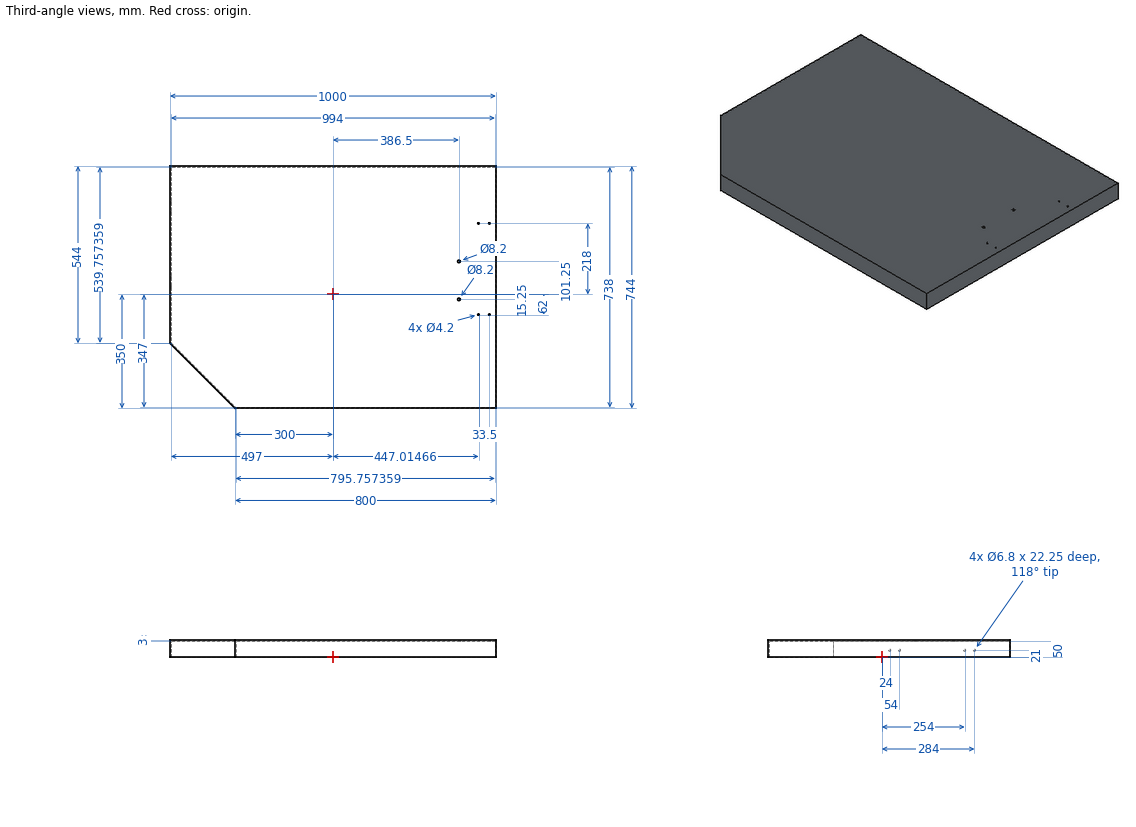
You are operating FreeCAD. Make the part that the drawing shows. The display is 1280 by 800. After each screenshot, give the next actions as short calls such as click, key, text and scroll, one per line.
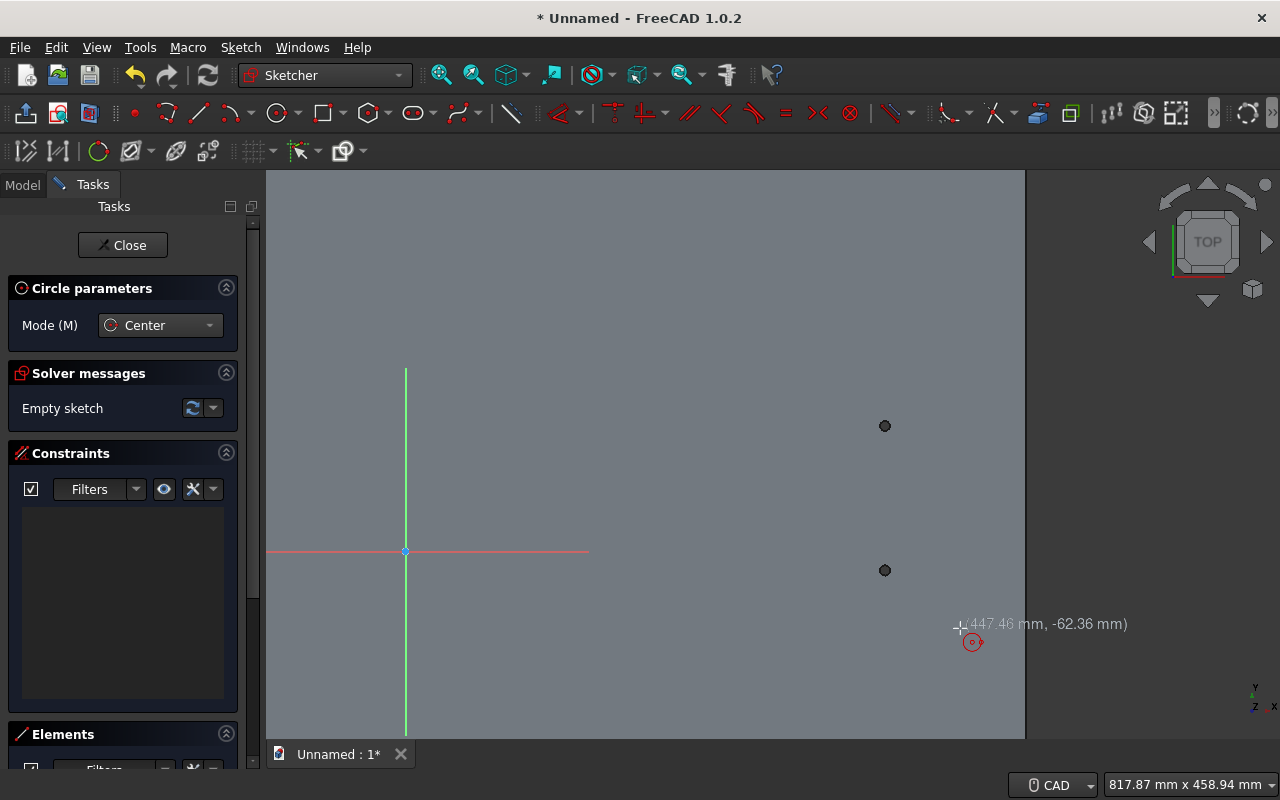
click(960, 628)
move(962, 627)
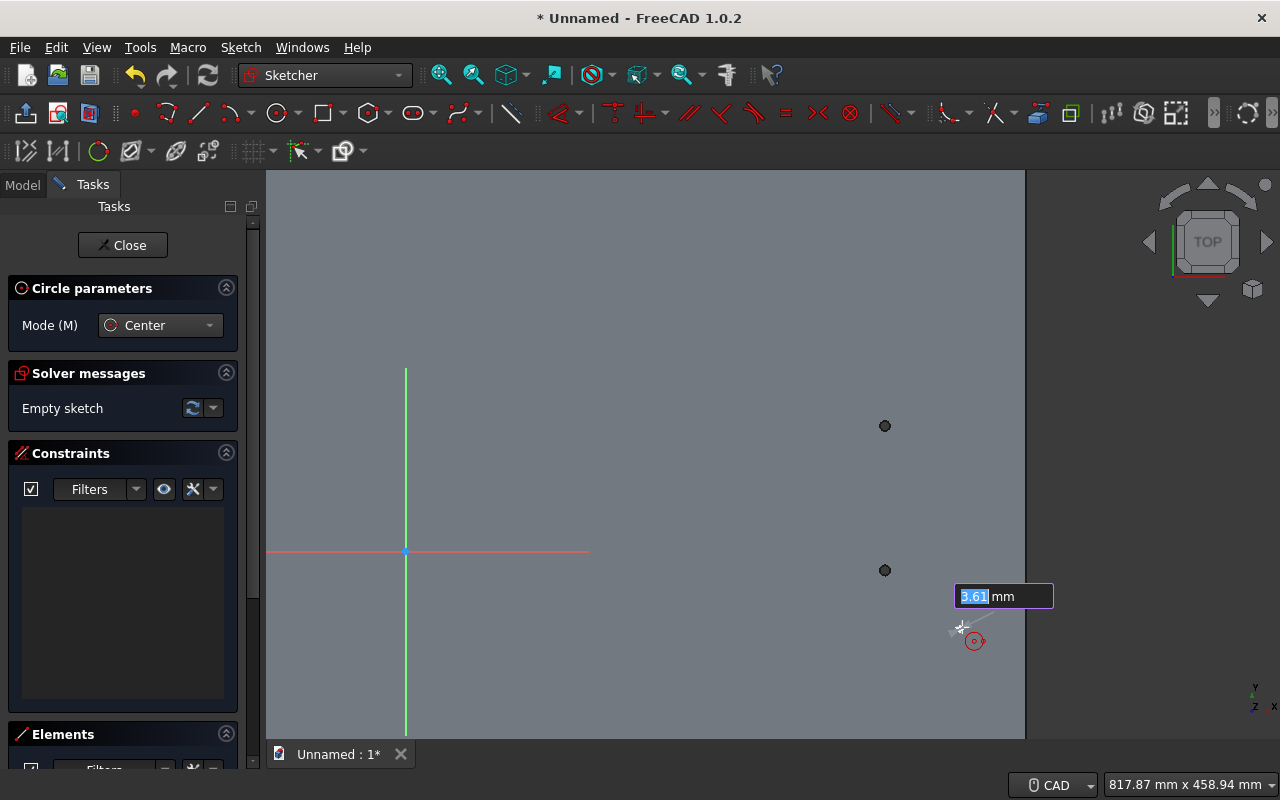
text(4.2)
key(Return)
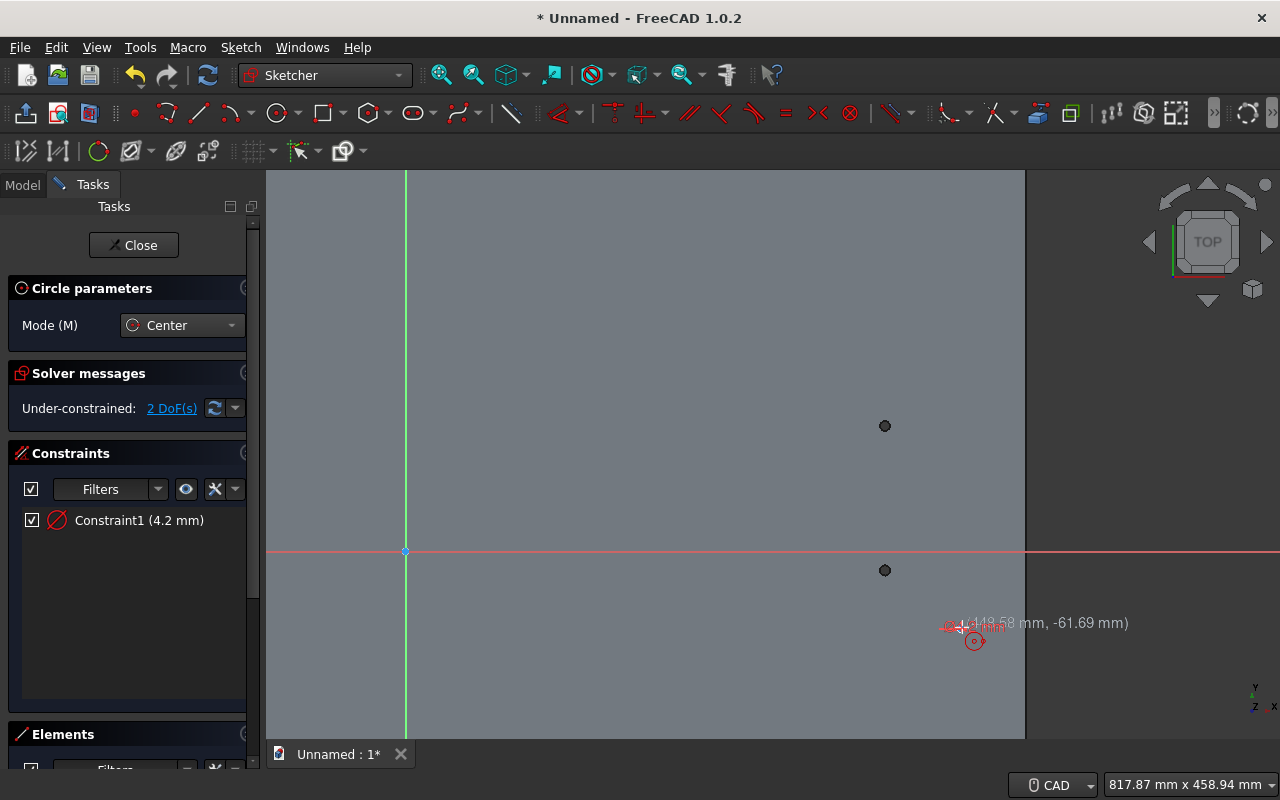
scroll(1002, 628, up, 11)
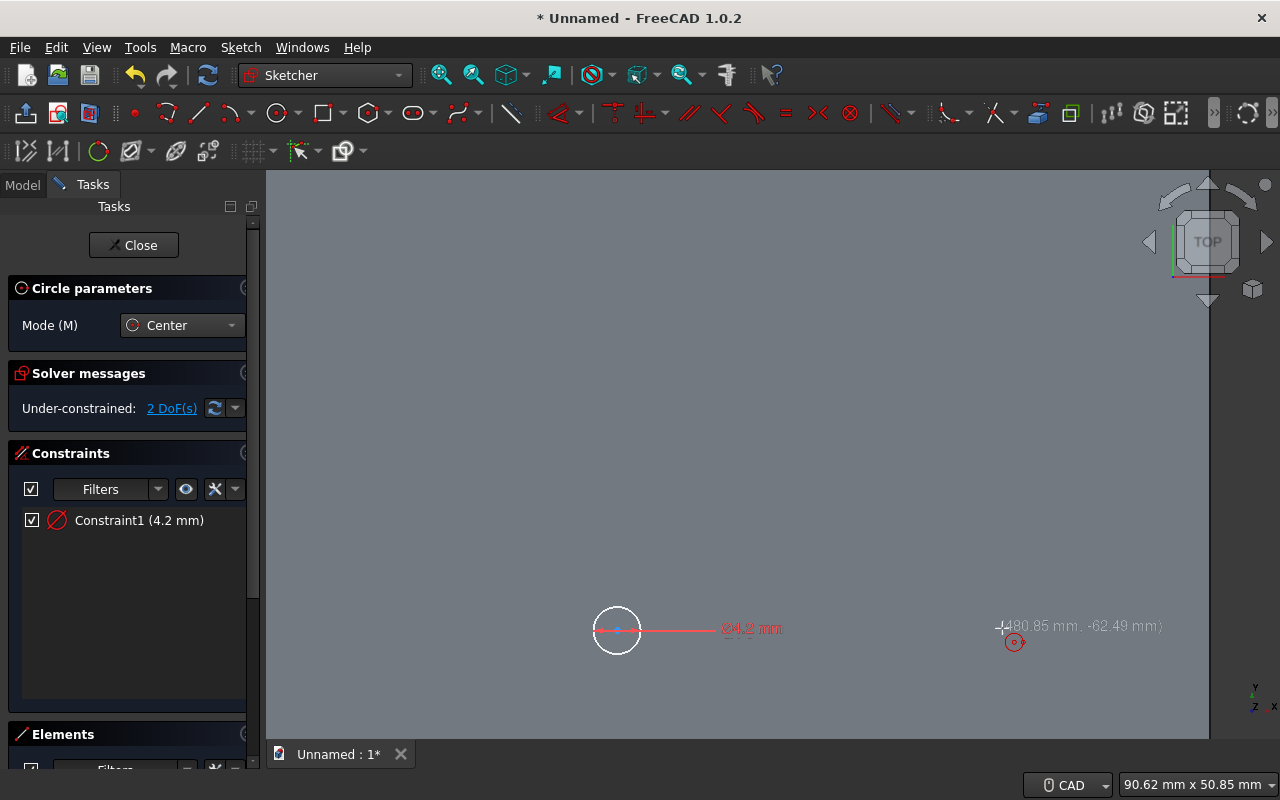
scroll(1002, 628, down, 11)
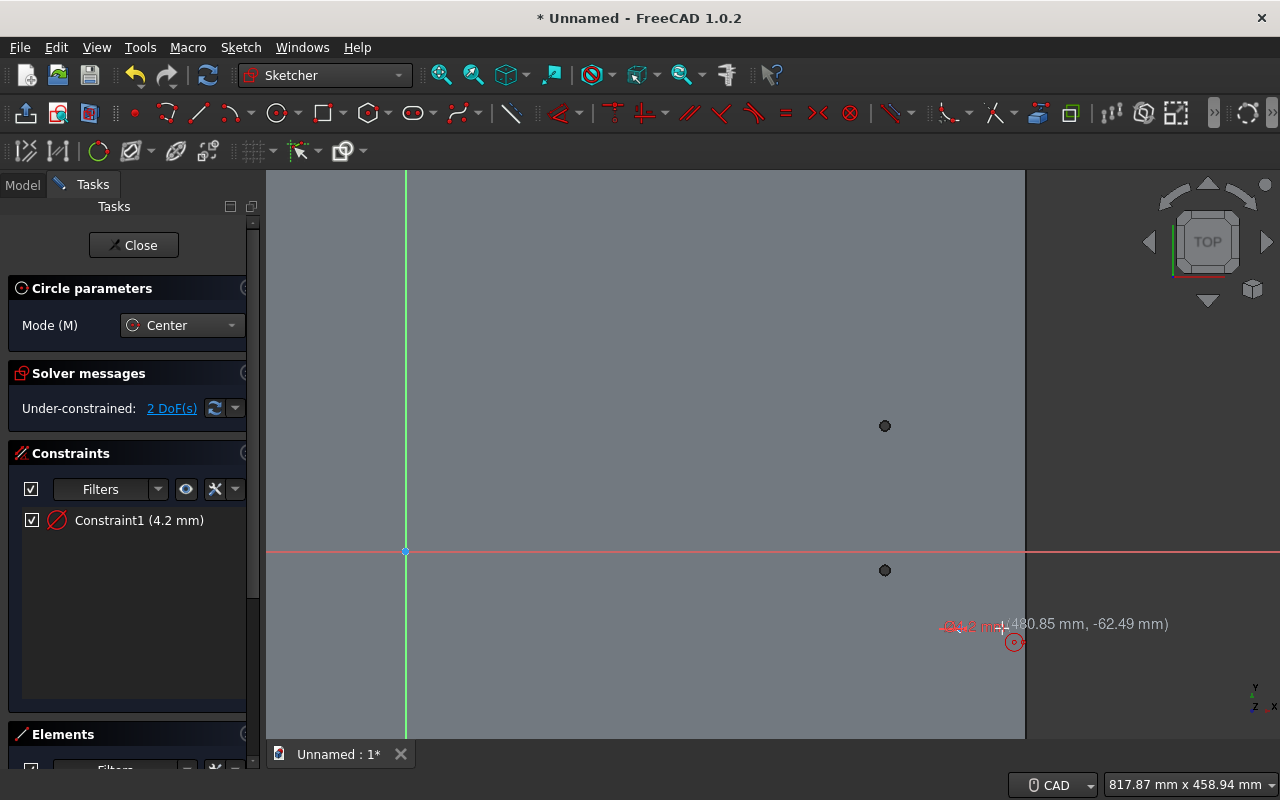
click(1002, 628)
move(1003, 627)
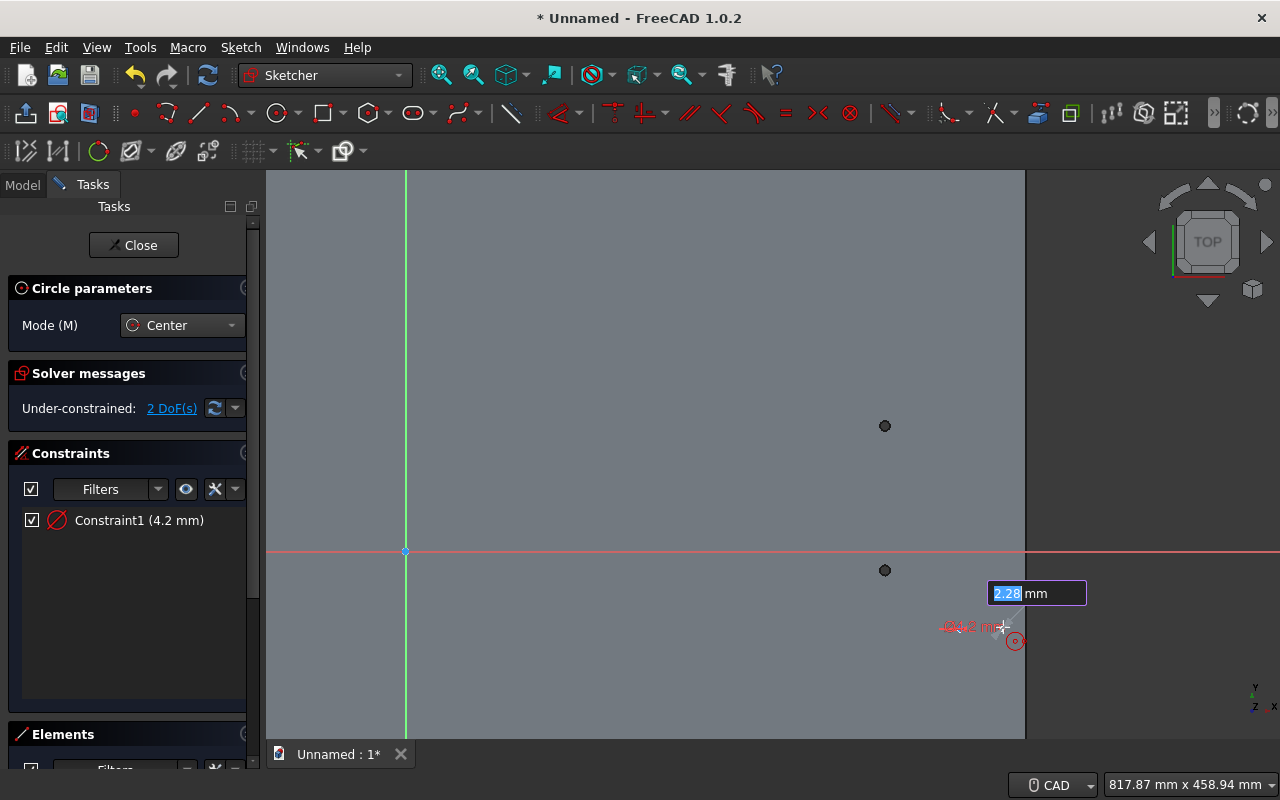
text(4.2)
key(Return)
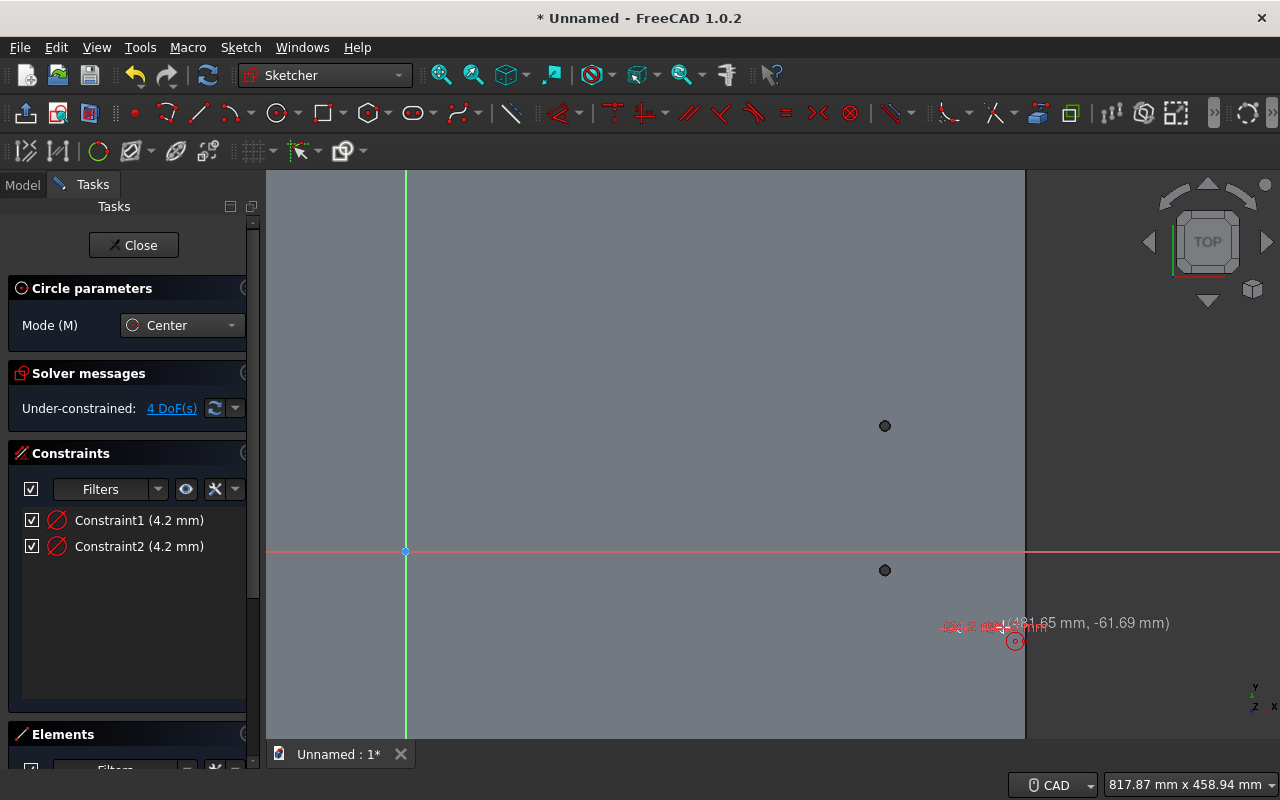
scroll(960, 281, up, 11)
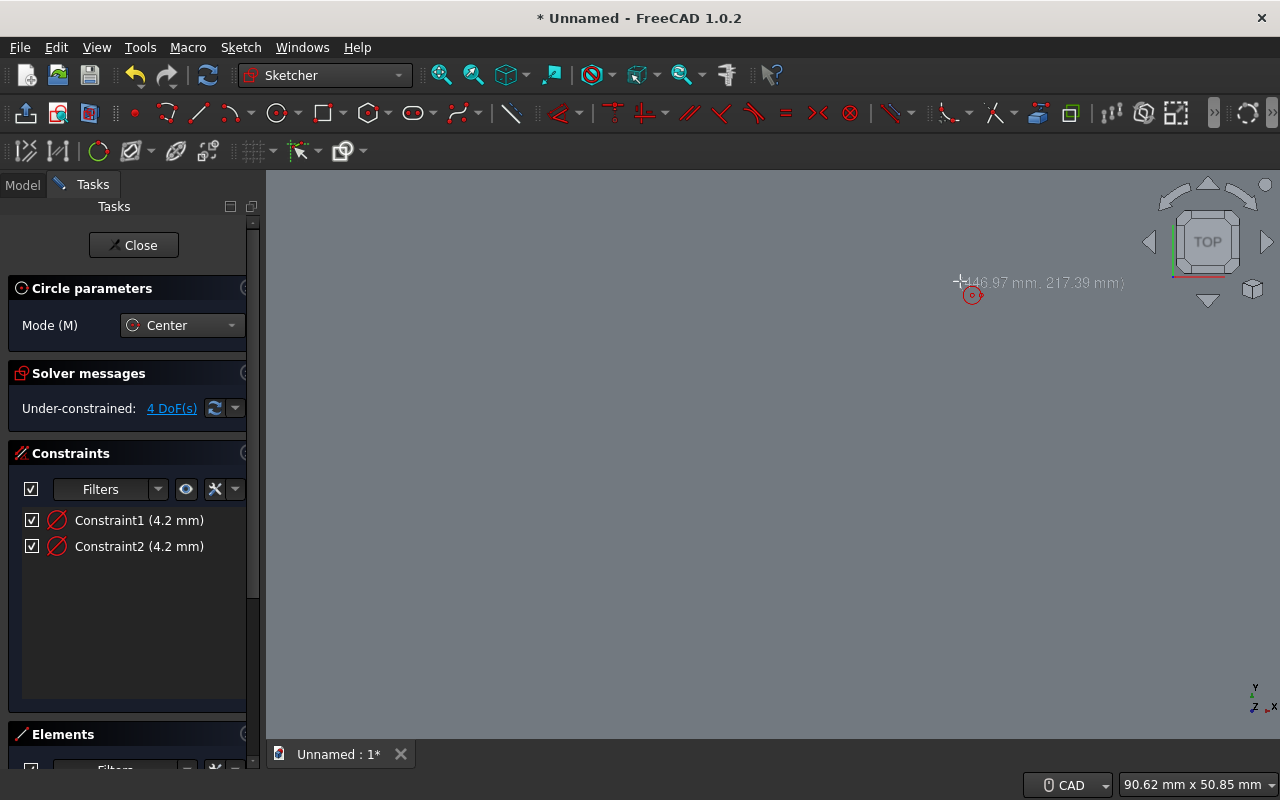
scroll(960, 281, down, 11)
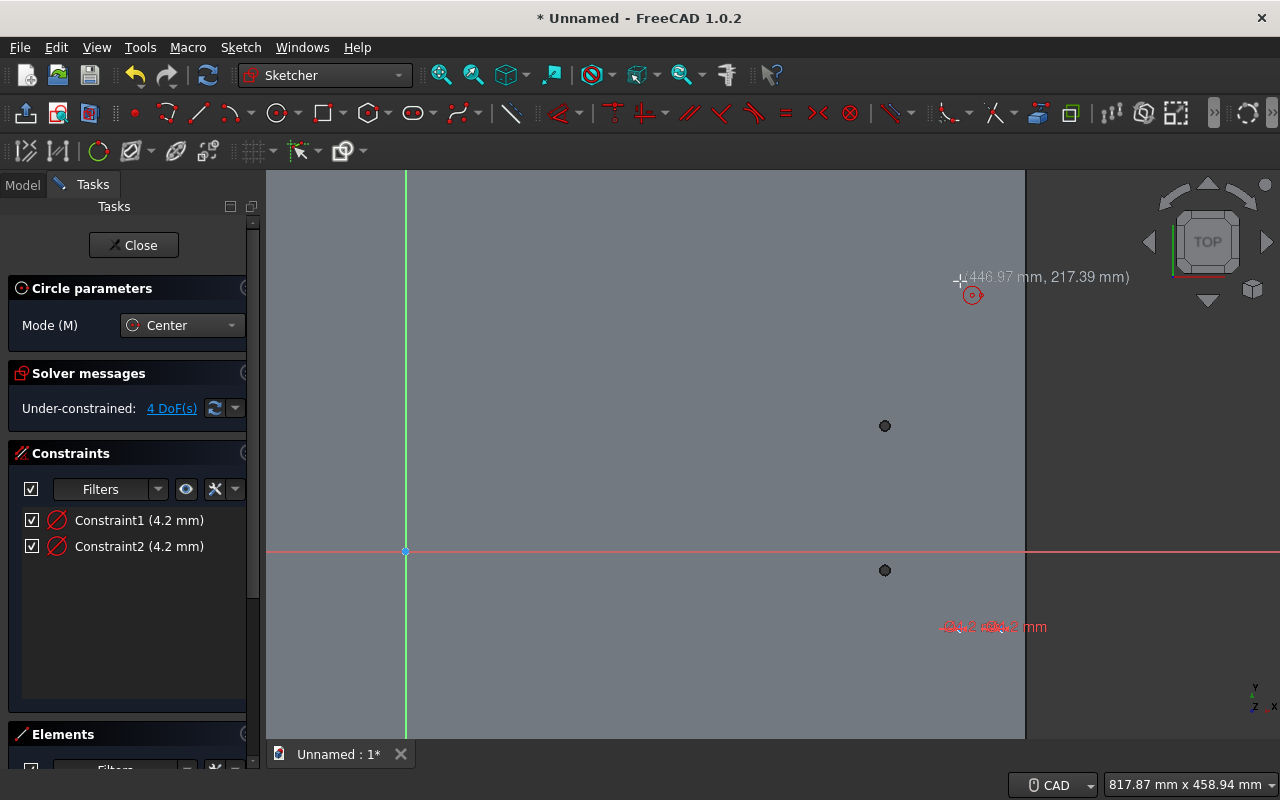
click(960, 281)
move(962, 279)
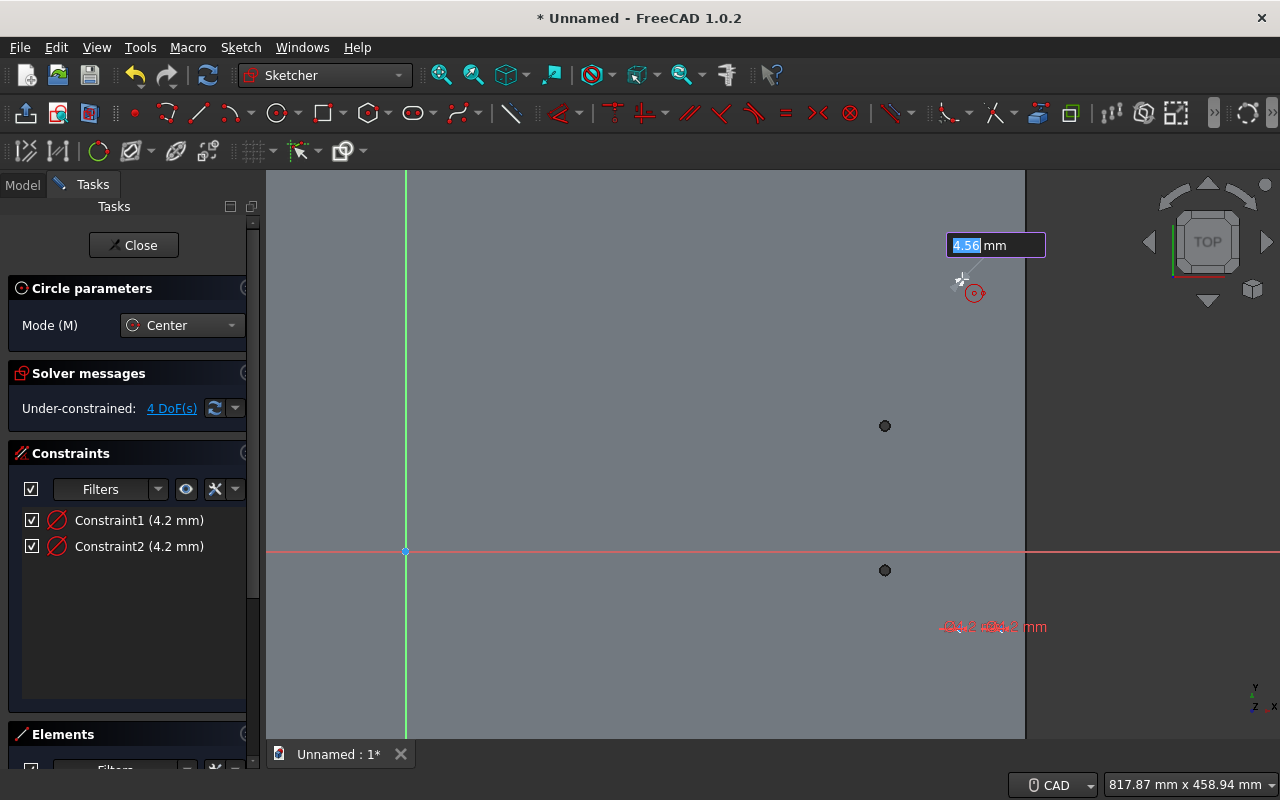
text(4.2)
key(Return)